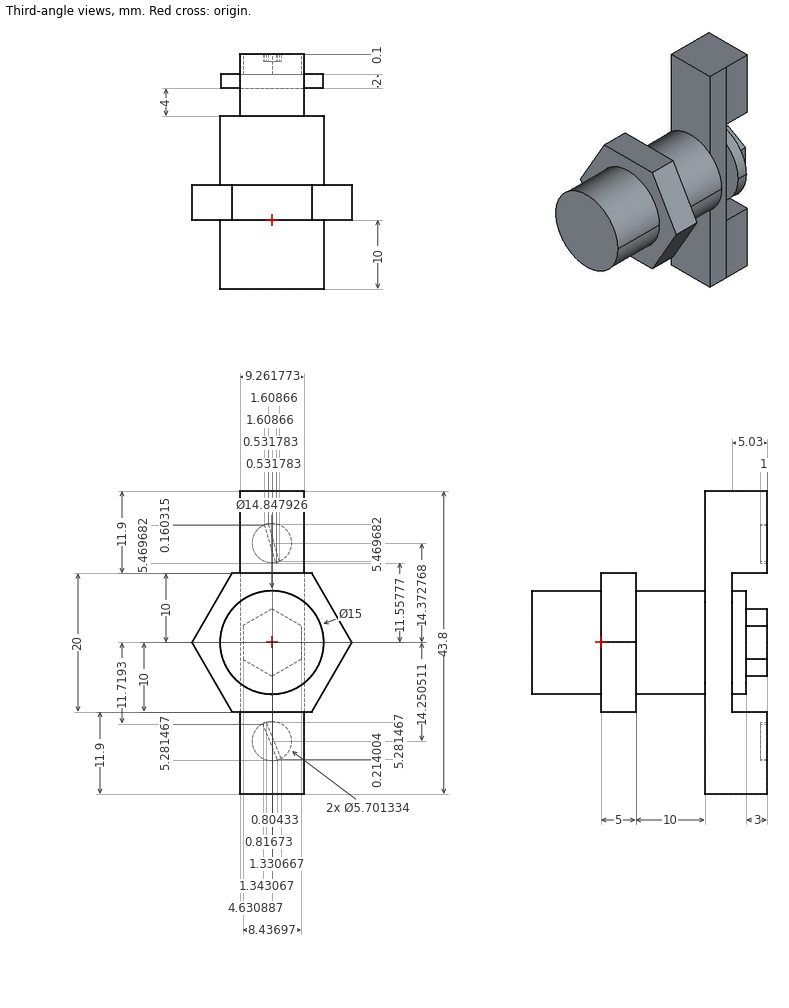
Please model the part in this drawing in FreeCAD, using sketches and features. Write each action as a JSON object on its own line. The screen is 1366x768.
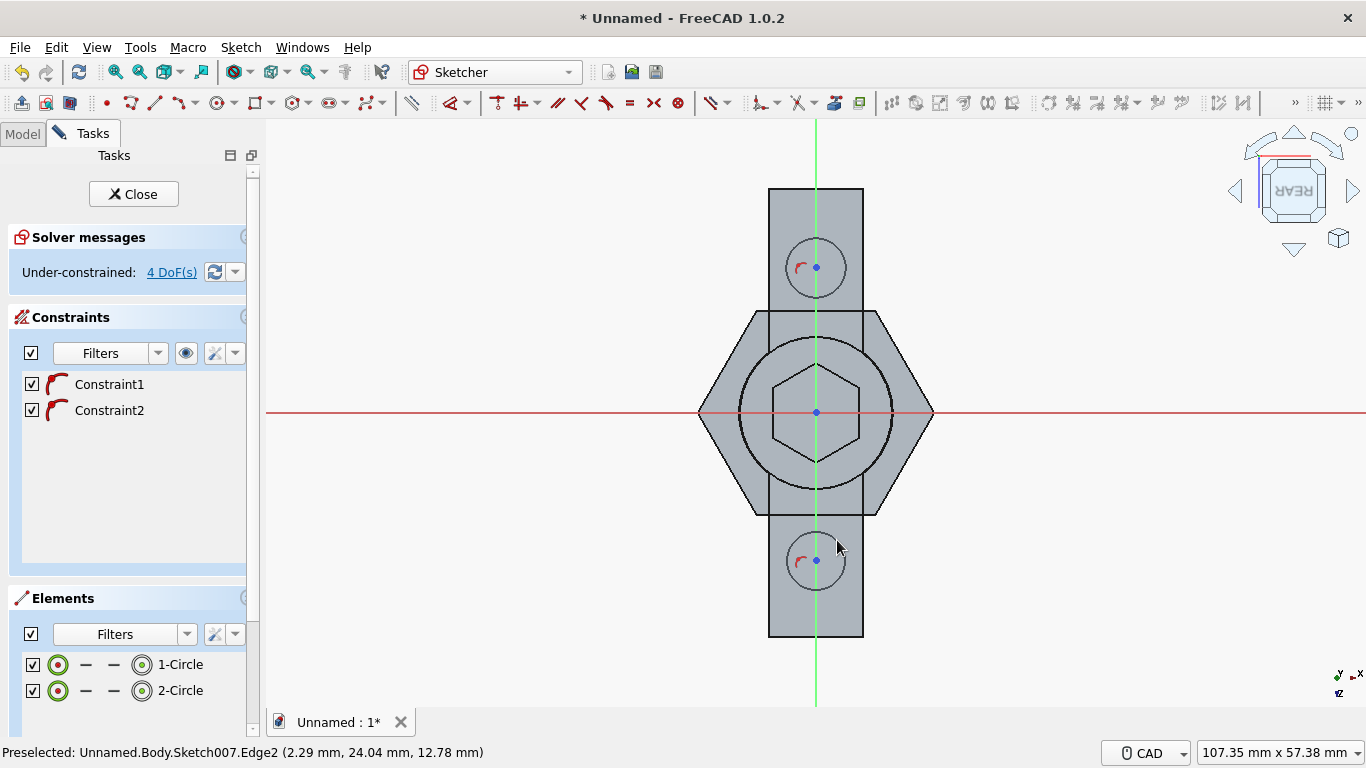
{"action": "left_click", "coordinate": [837, 247]}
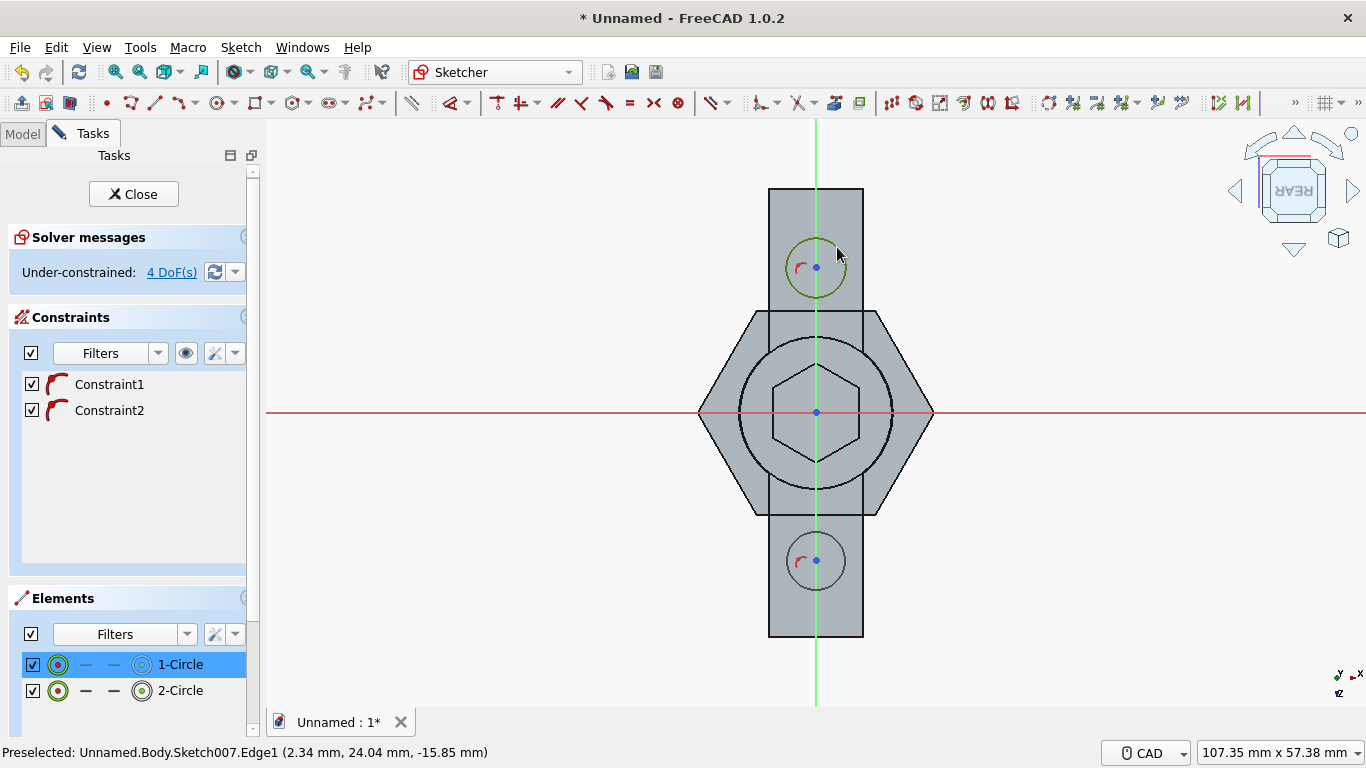
{"action": "left_click", "coordinate": [836, 540]}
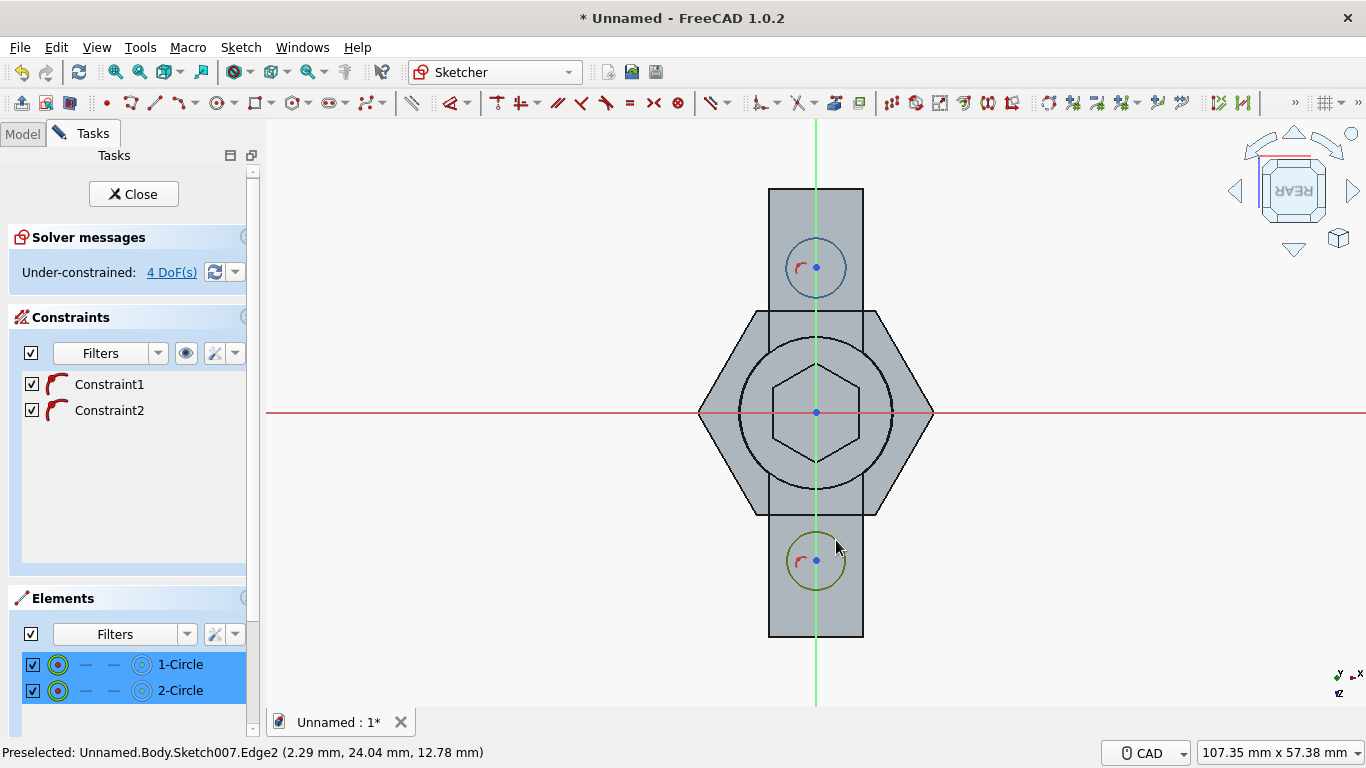
{"action": "left_click", "coordinate": [630, 104]}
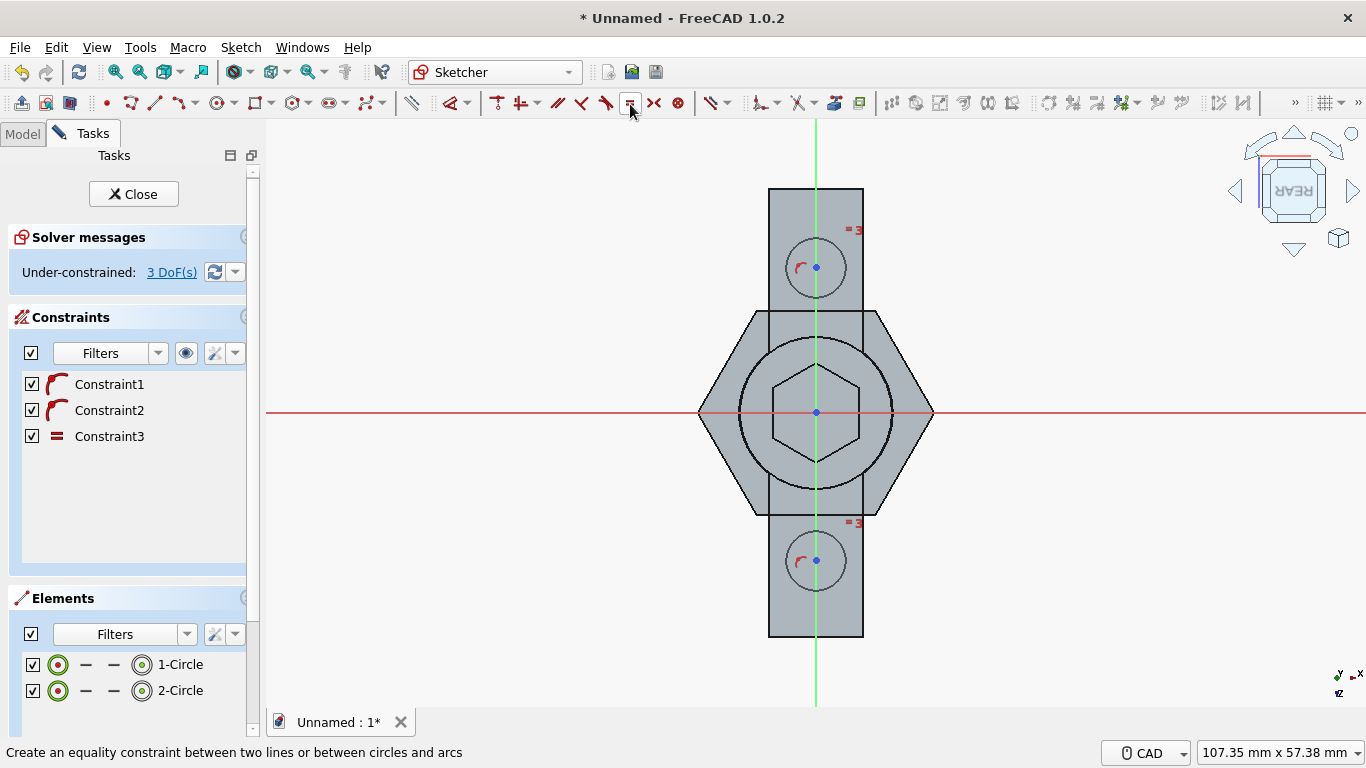
{"action": "left_click", "coordinate": [450, 104]}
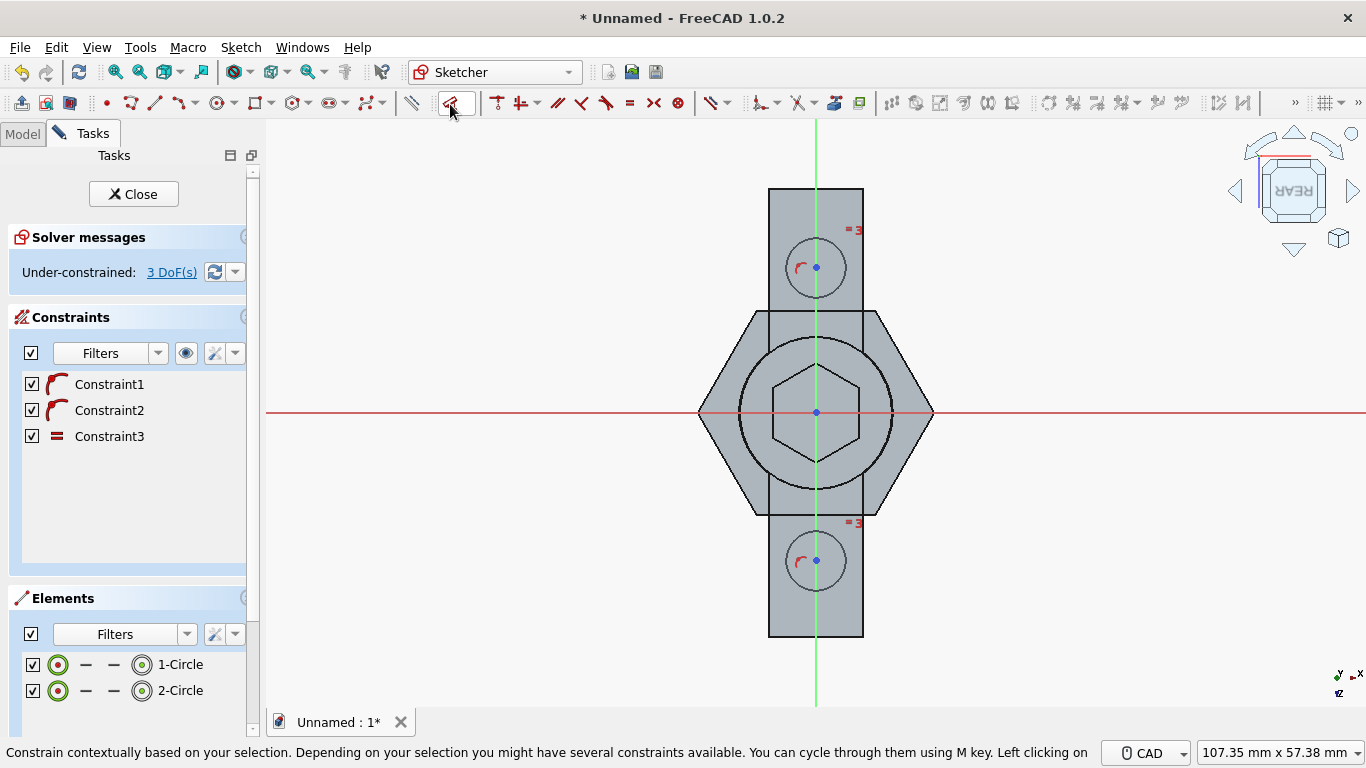
{"action": "left_click", "coordinate": [837, 247]}
{"action": "left_click", "coordinate": [860, 224]}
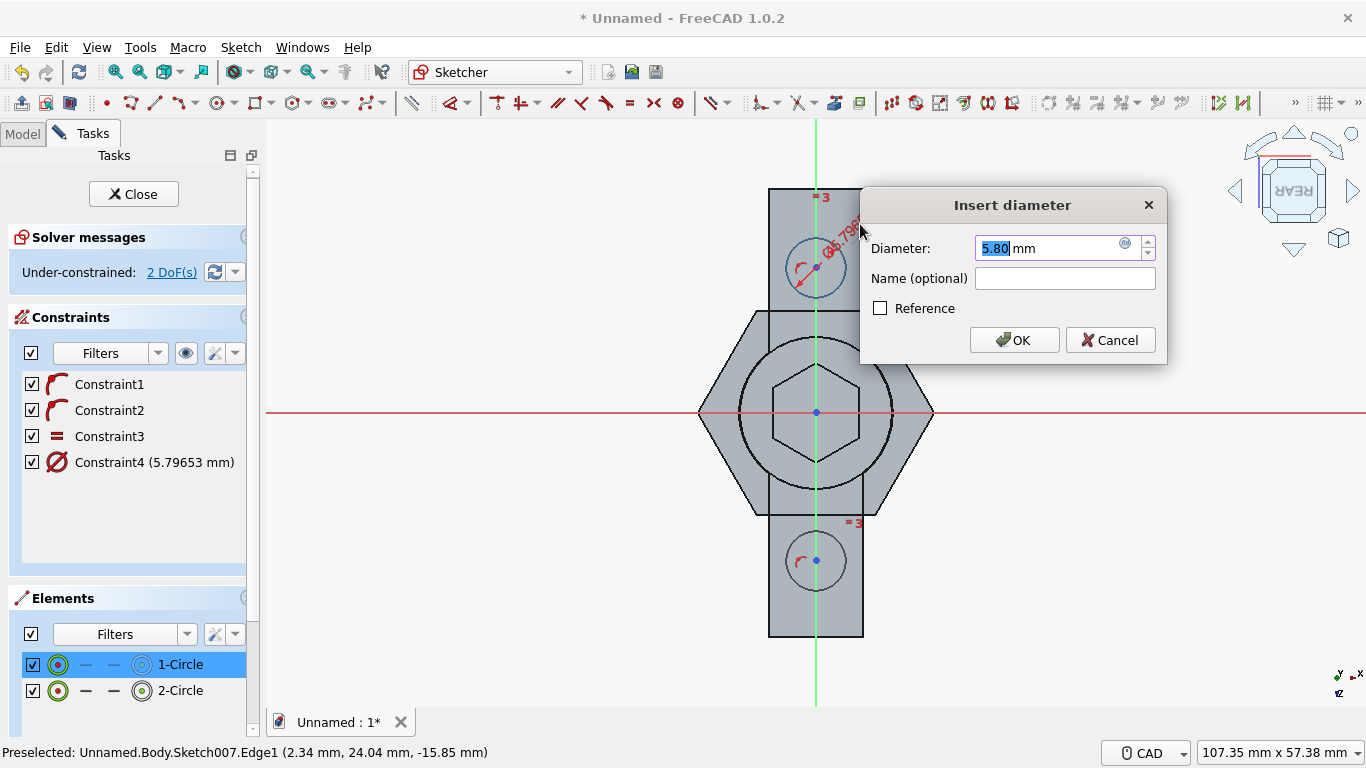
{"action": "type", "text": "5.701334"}
{"action": "key", "text": "Return"}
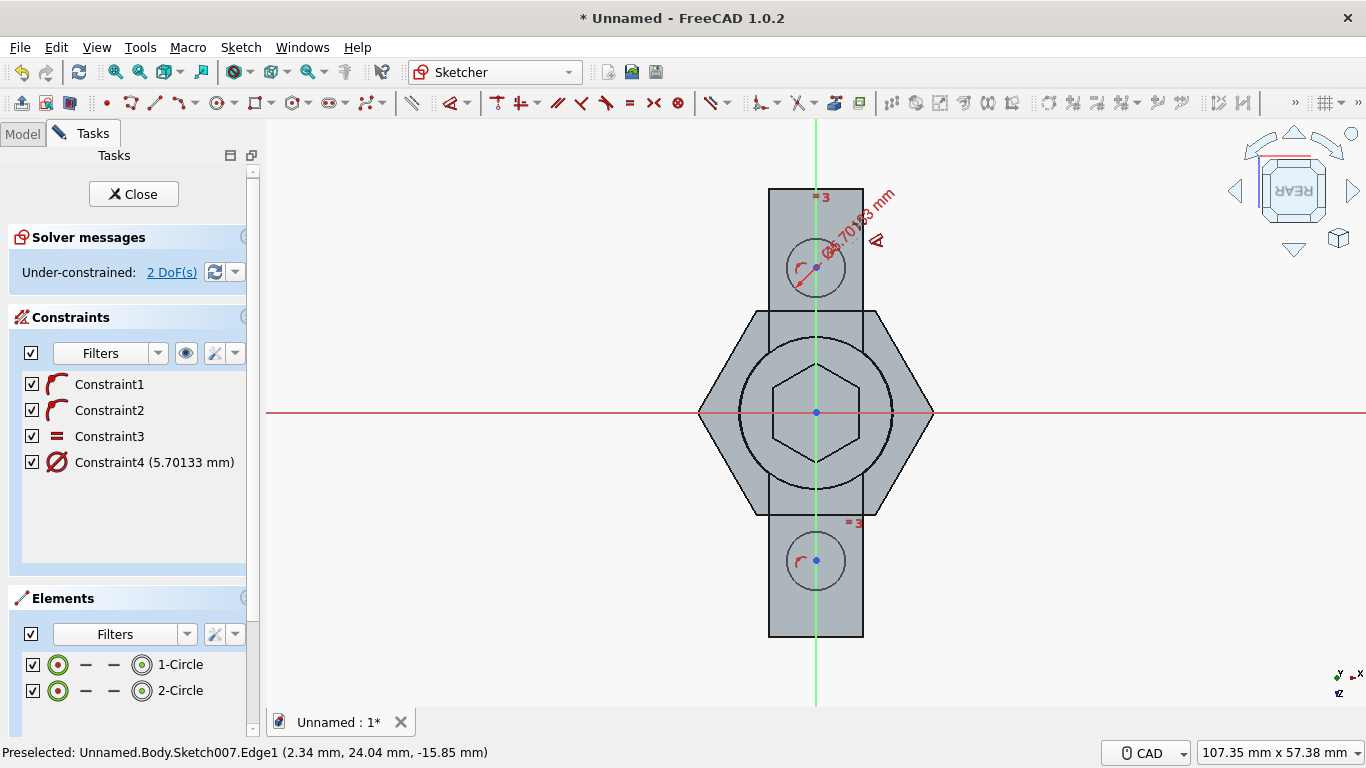
{"action": "left_click", "coordinate": [816, 268]}
{"action": "left_click", "coordinate": [850, 341]}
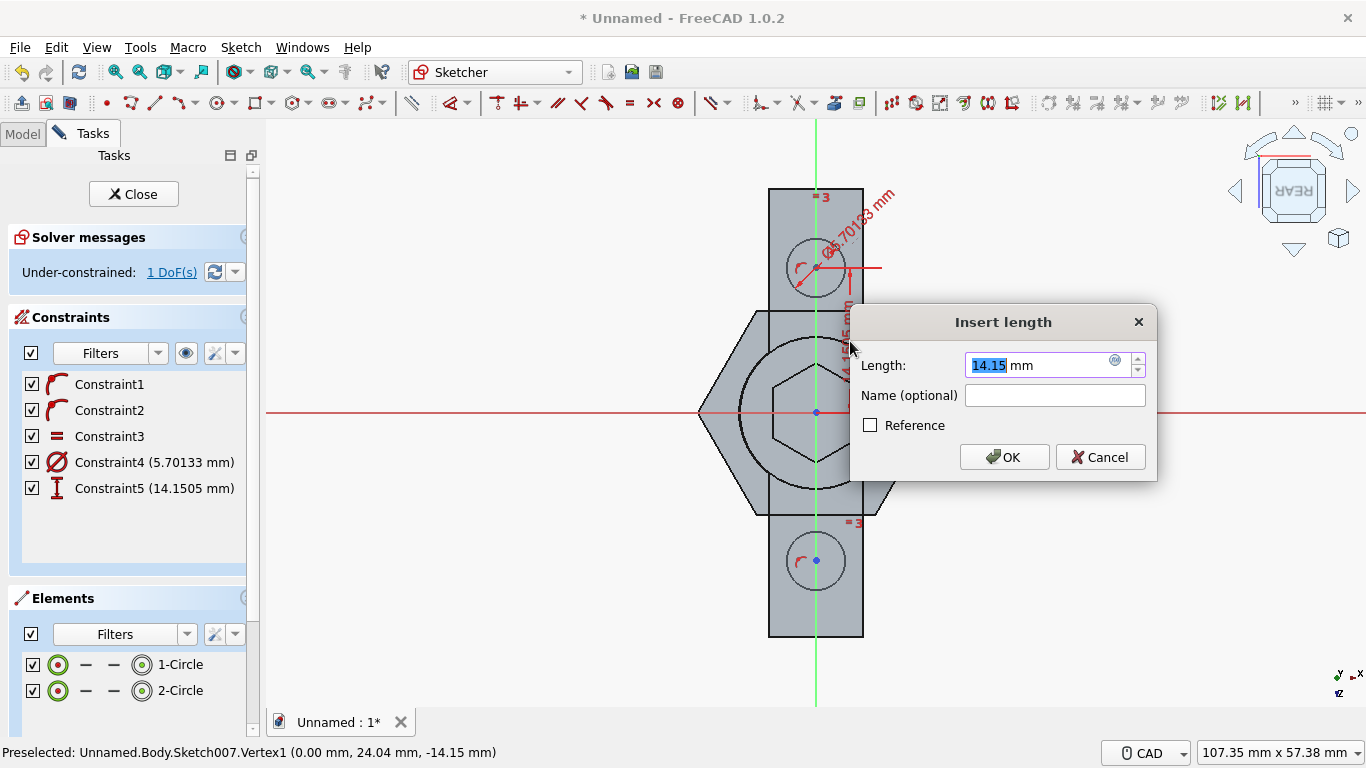
{"action": "type", "text": "14.250511"}
{"action": "key", "text": "Return"}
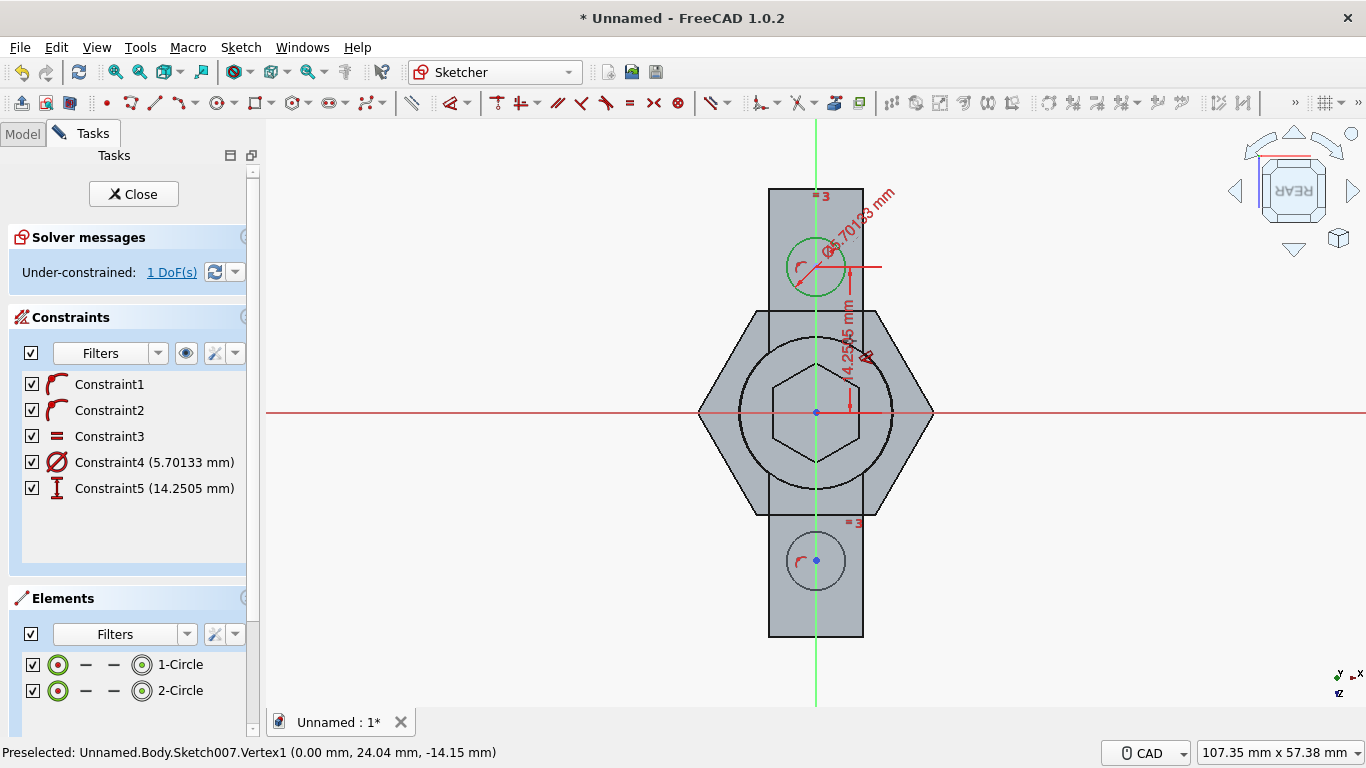
{"action": "left_click", "coordinate": [816, 561]}
{"action": "left_click", "coordinate": [850, 487]}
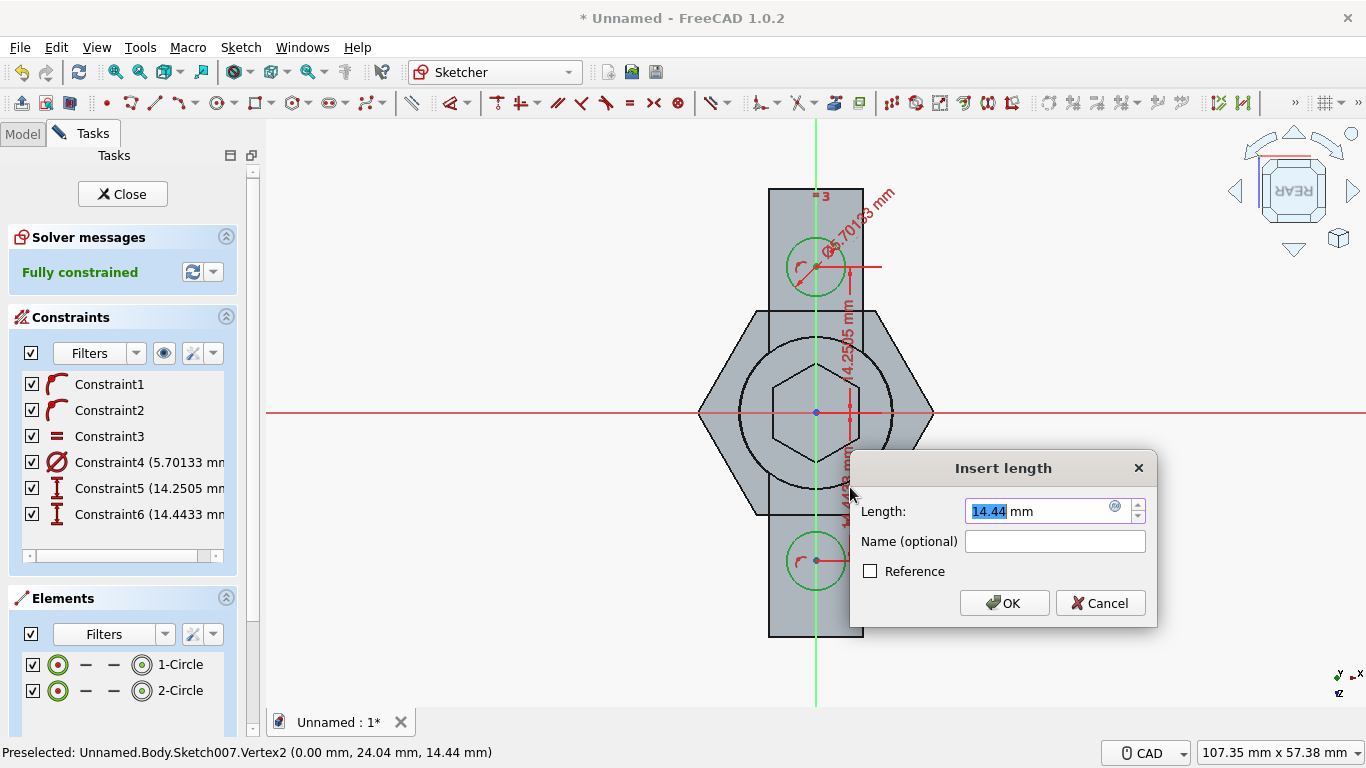
{"action": "type", "text": "14.372768"}
{"action": "key", "text": "Return"}
{"action": "key", "text": "Escape"}